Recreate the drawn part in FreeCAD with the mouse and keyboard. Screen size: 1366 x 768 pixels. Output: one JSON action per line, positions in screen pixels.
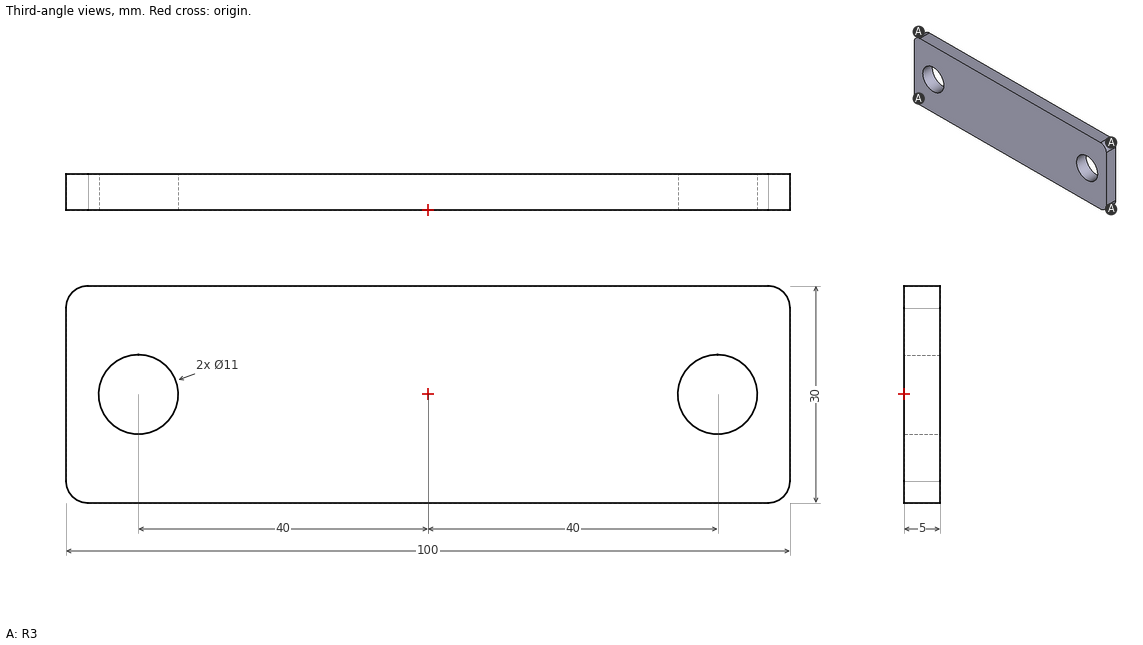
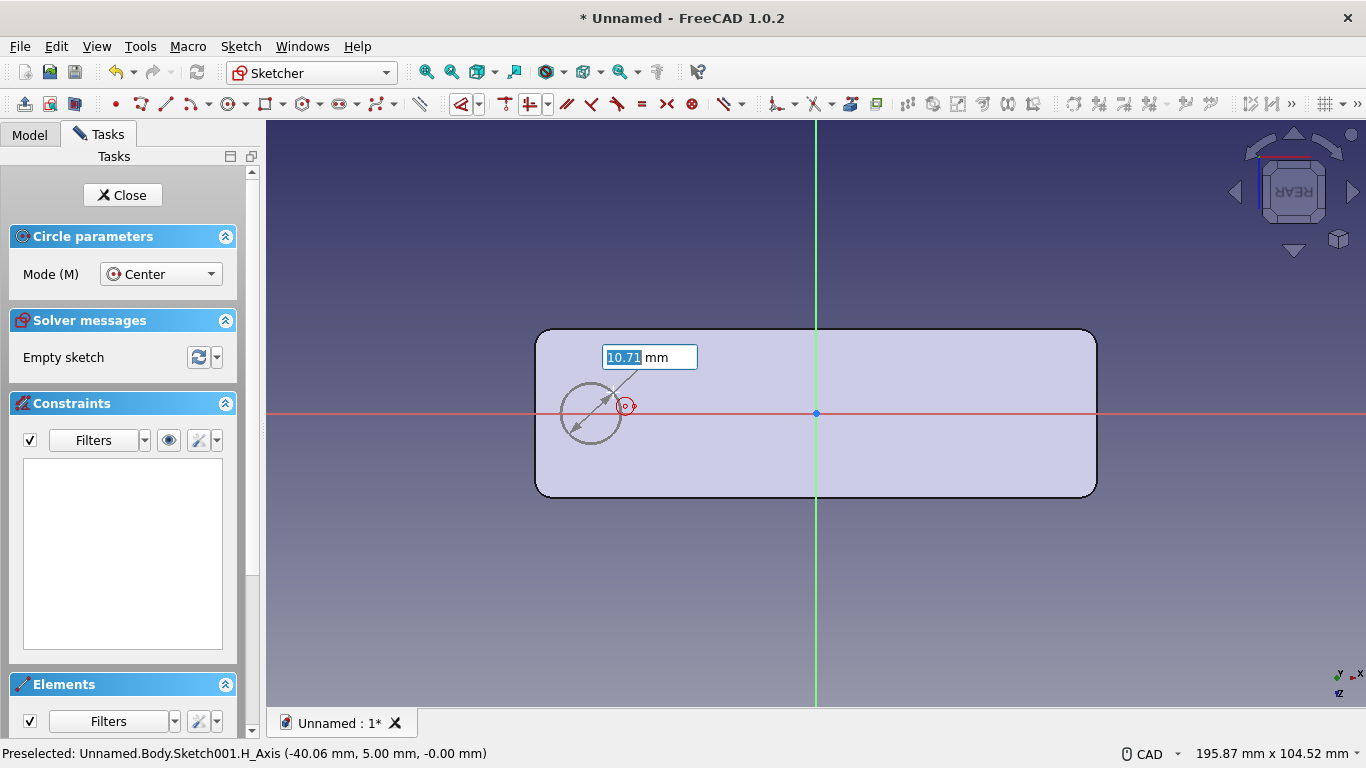
{"action": "type", "text": "11"}
{"action": "key", "text": "Return"}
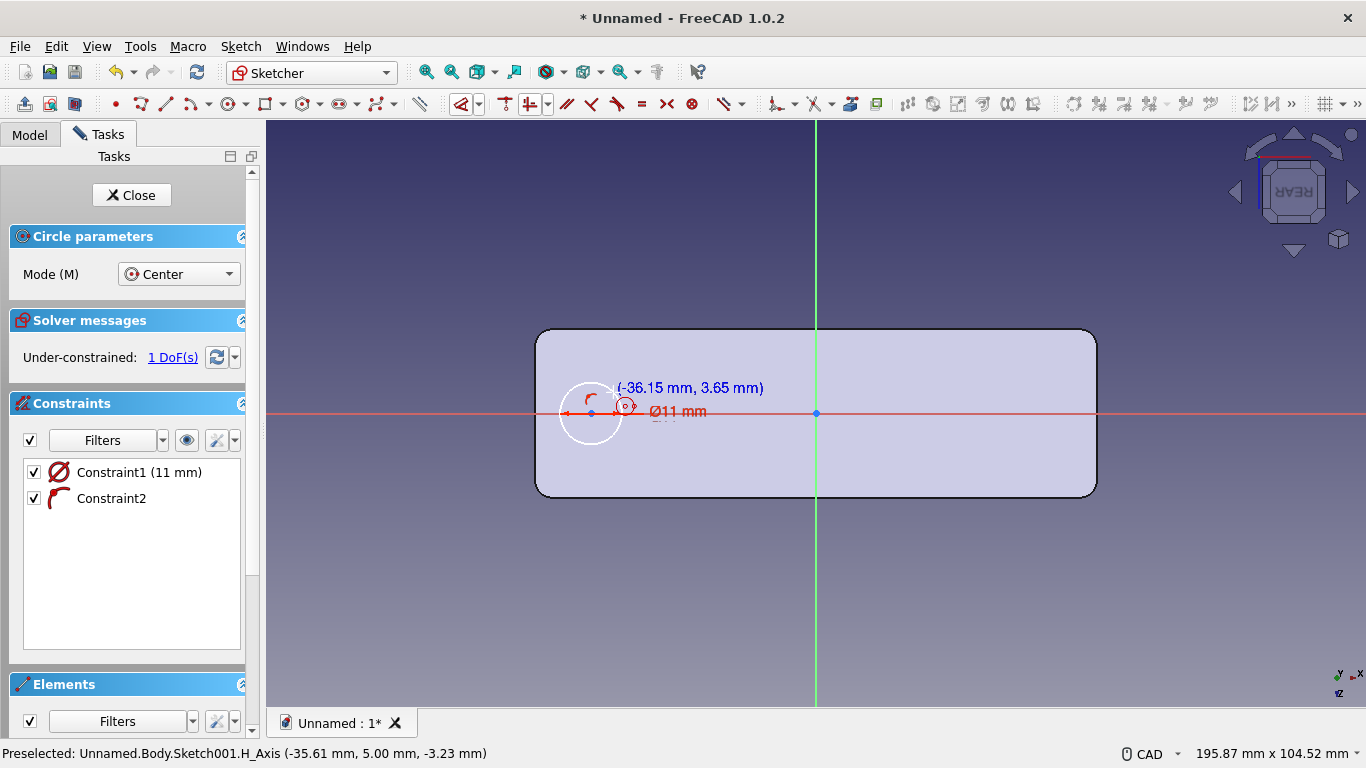
{"action": "left_click", "coordinate": [1041, 414]}
{"action": "mouse_move", "coordinate": [1062, 392]}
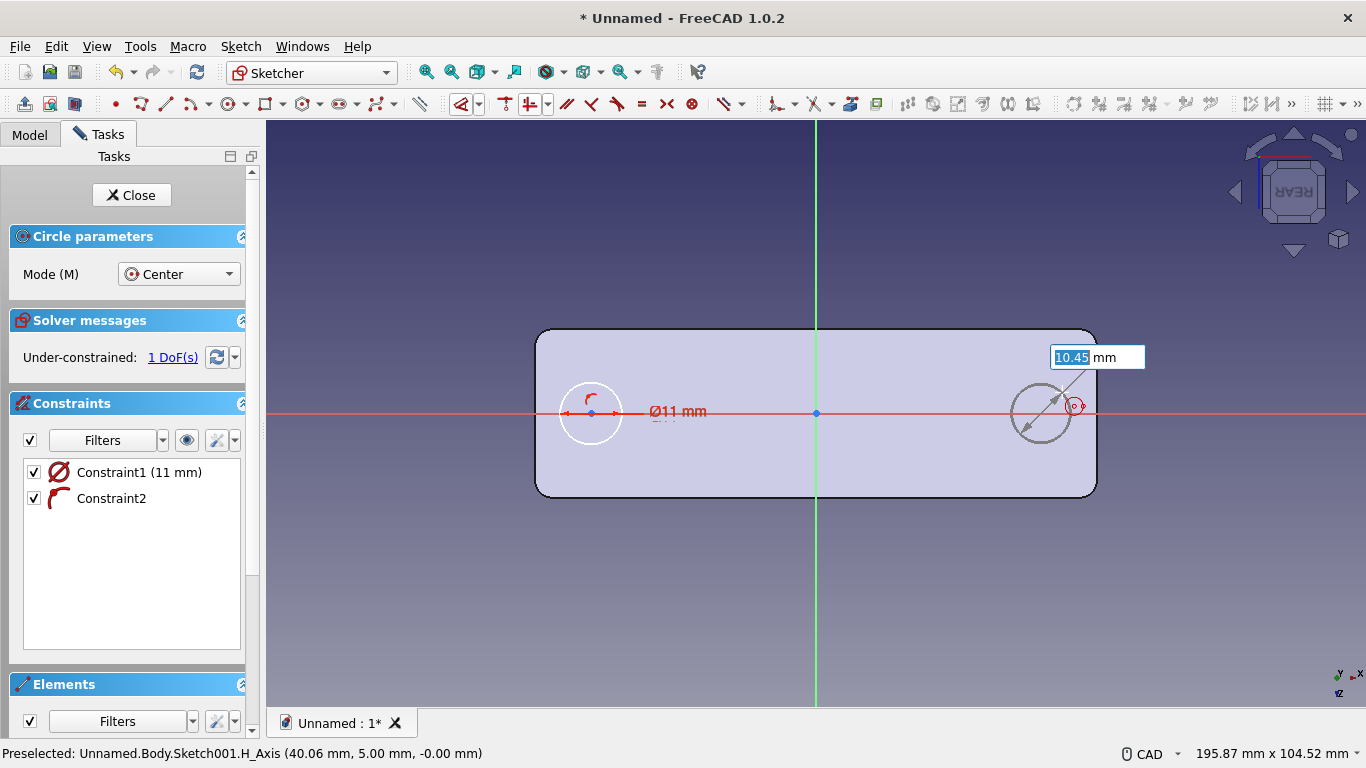
{"action": "type", "text": "11"}
{"action": "key", "text": "Return"}
{"action": "key", "text": "Escape"}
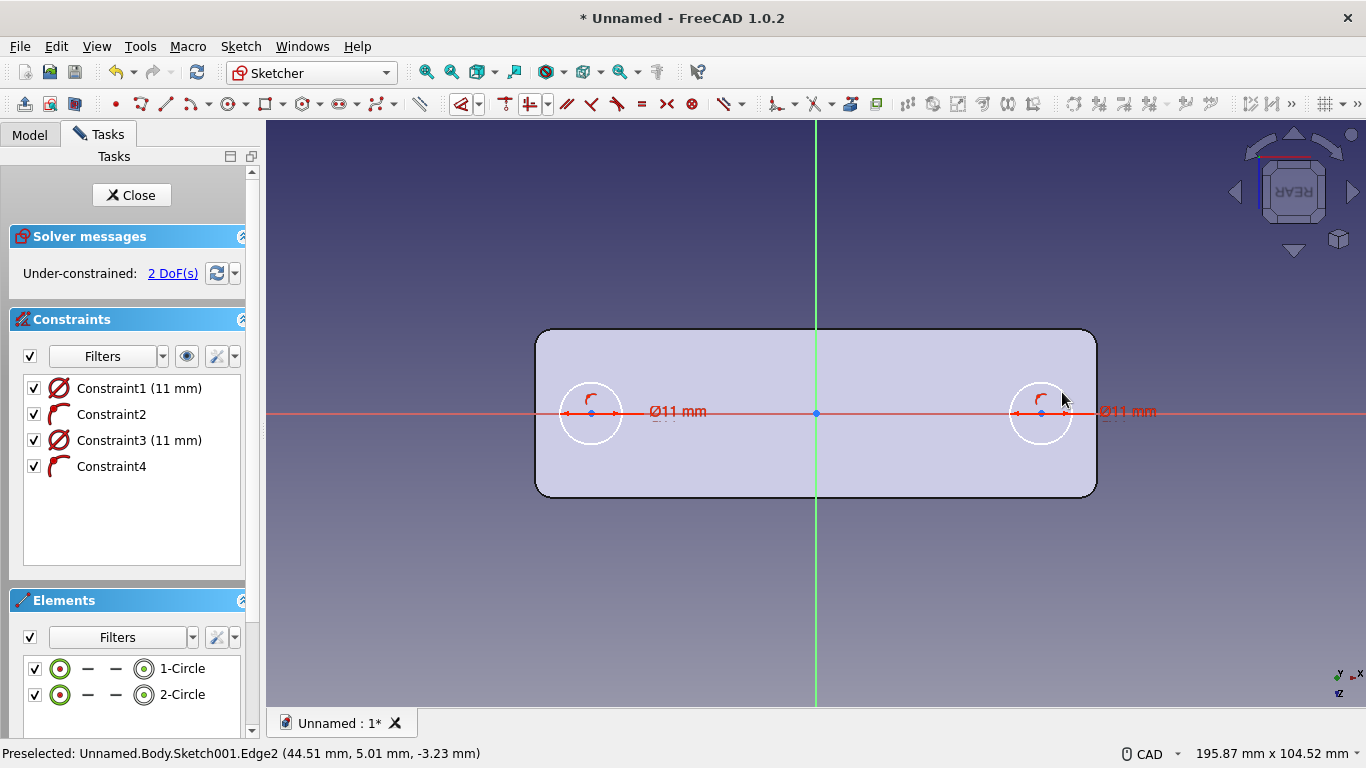
{"action": "key", "text": "d"}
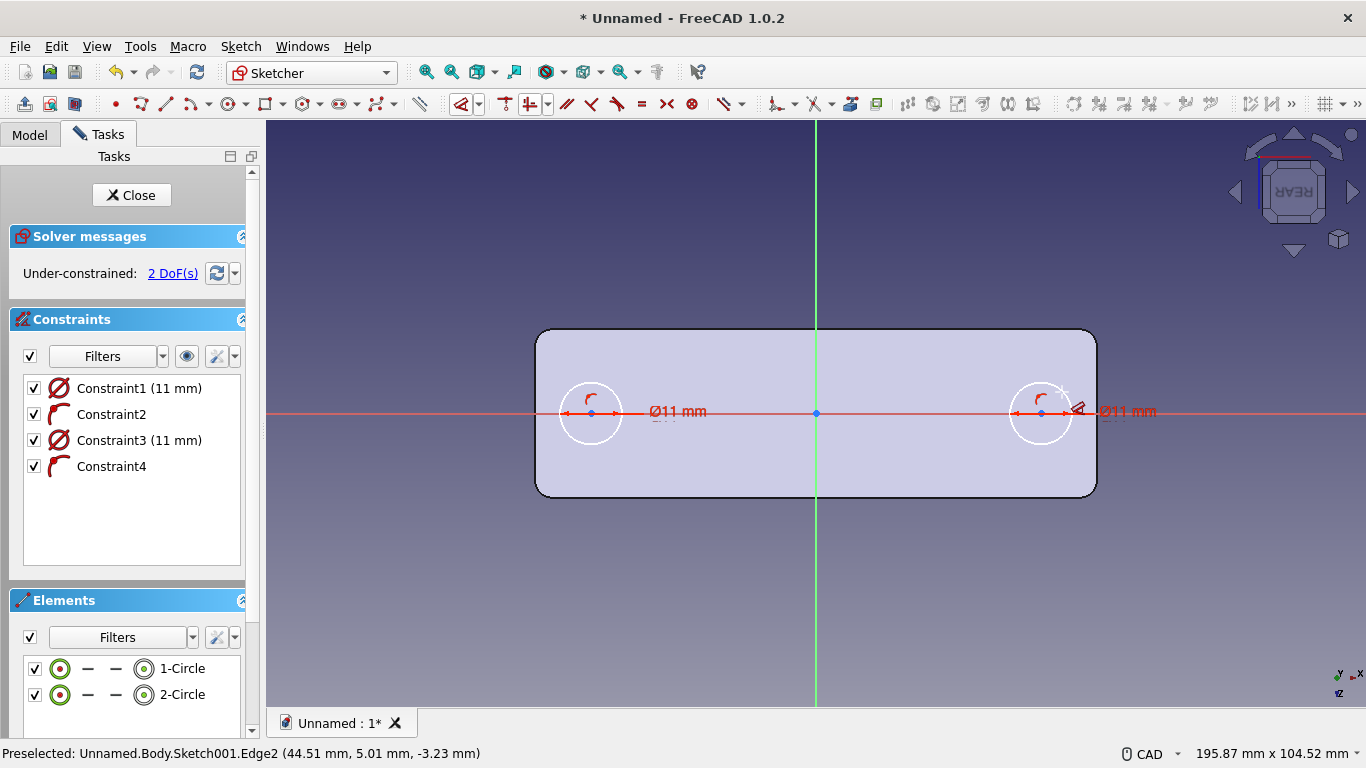
{"action": "left_click", "coordinate": [591, 414]}
{"action": "left_click", "coordinate": [703, 448]}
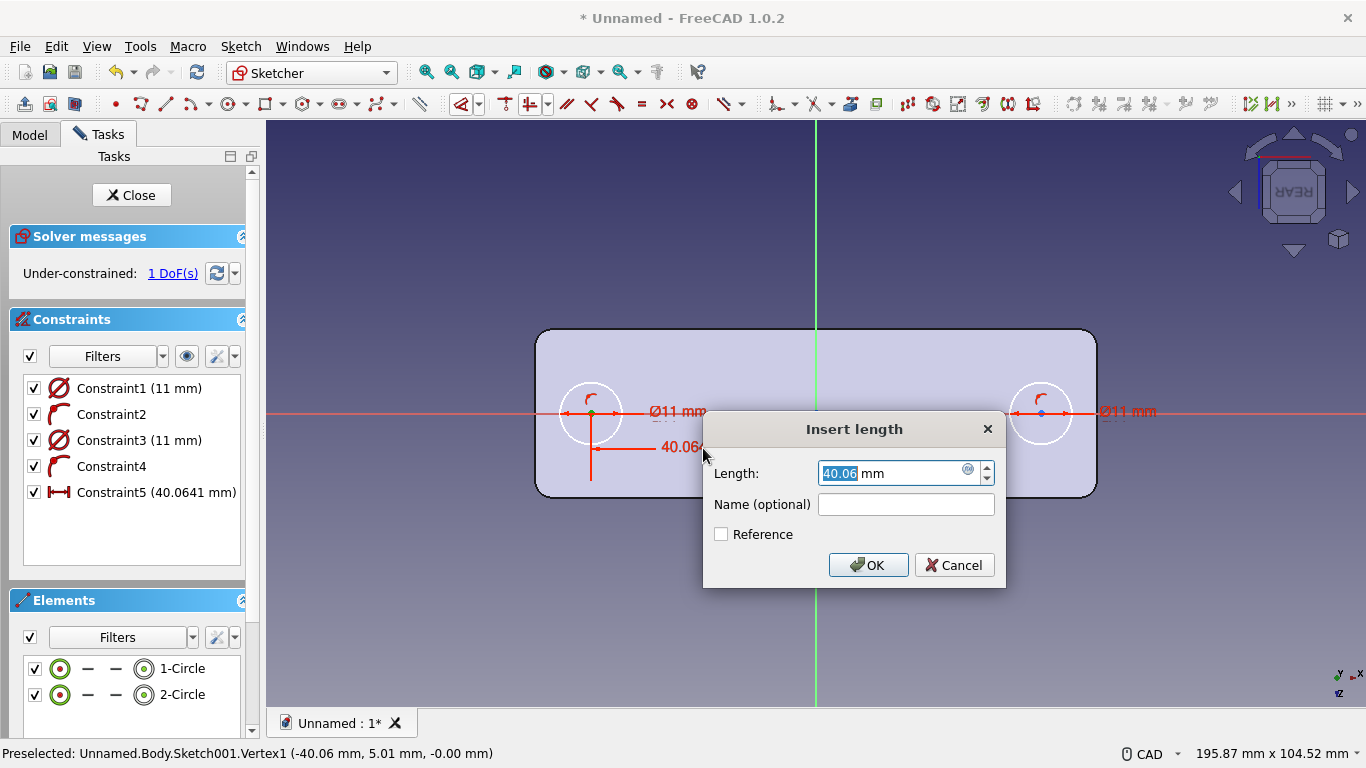
{"action": "type", "text": "40"}
{"action": "key", "text": "Return"}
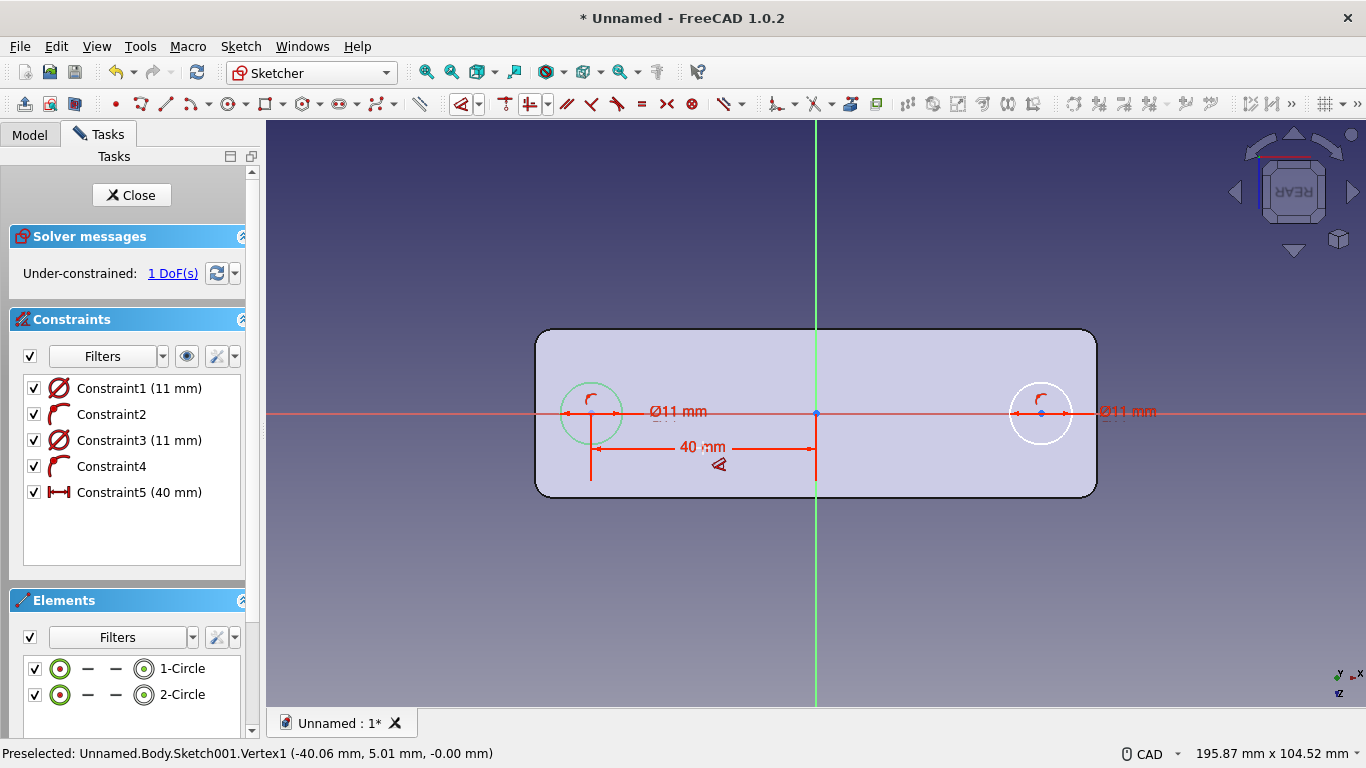
{"action": "left_click", "coordinate": [1041, 414]}
{"action": "left_click", "coordinate": [928, 448]}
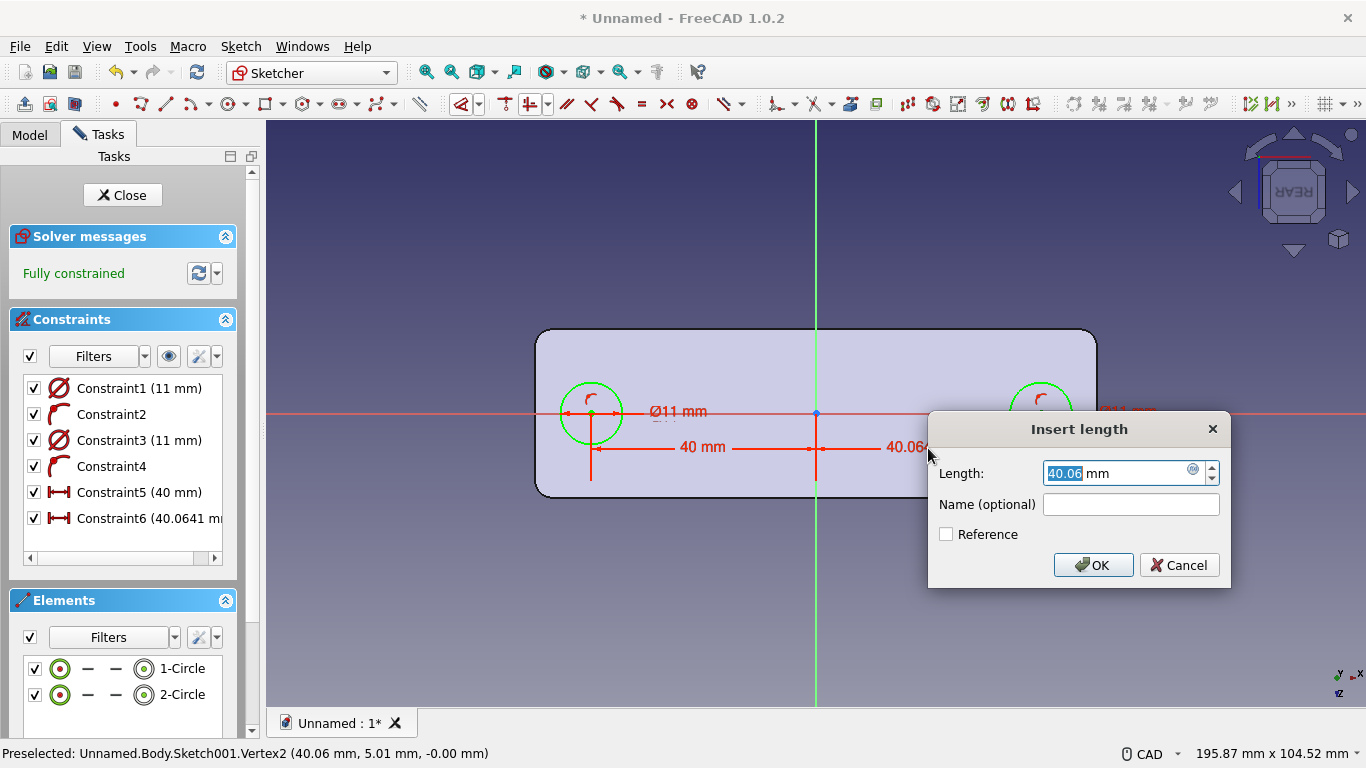
{"action": "type", "text": "40"}
{"action": "key", "text": "Return"}
{"action": "key", "text": "Escape"}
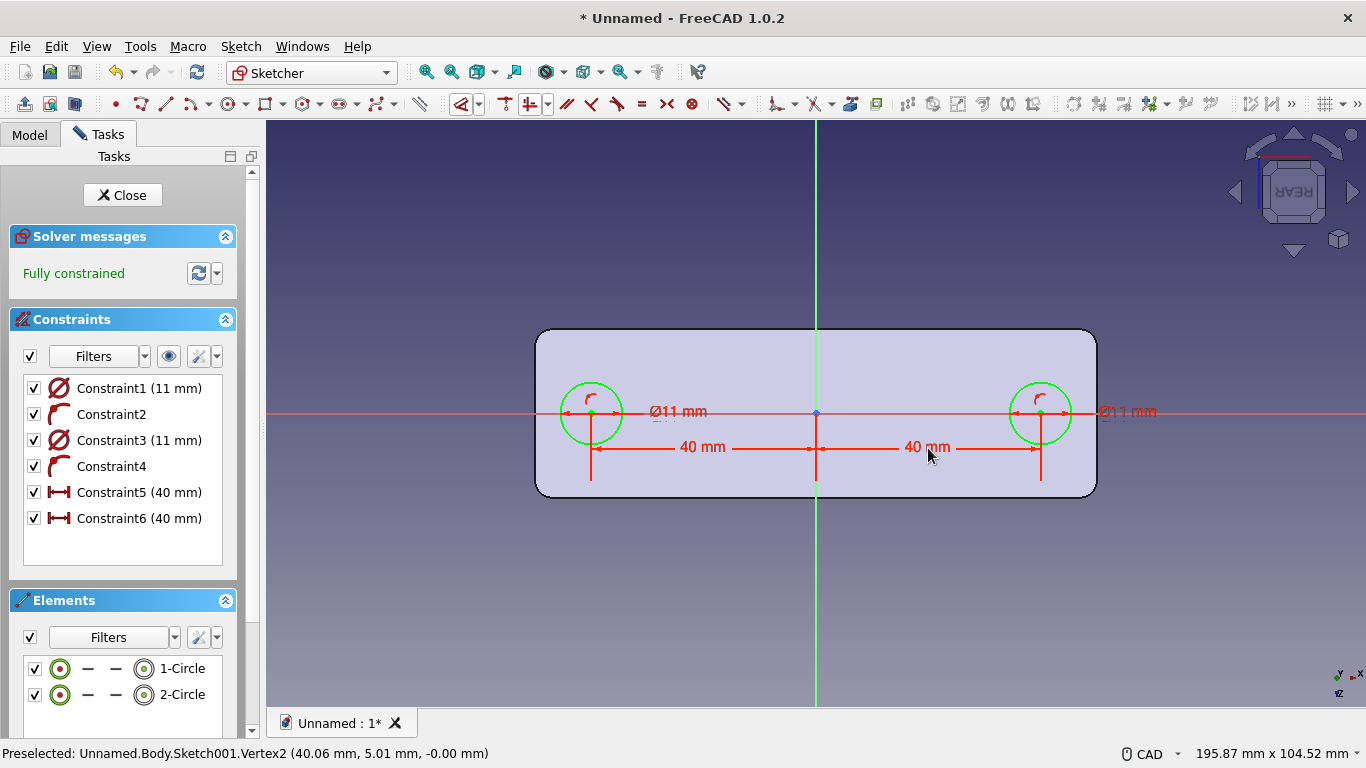
{"action": "left_click", "coordinate": [123, 195]}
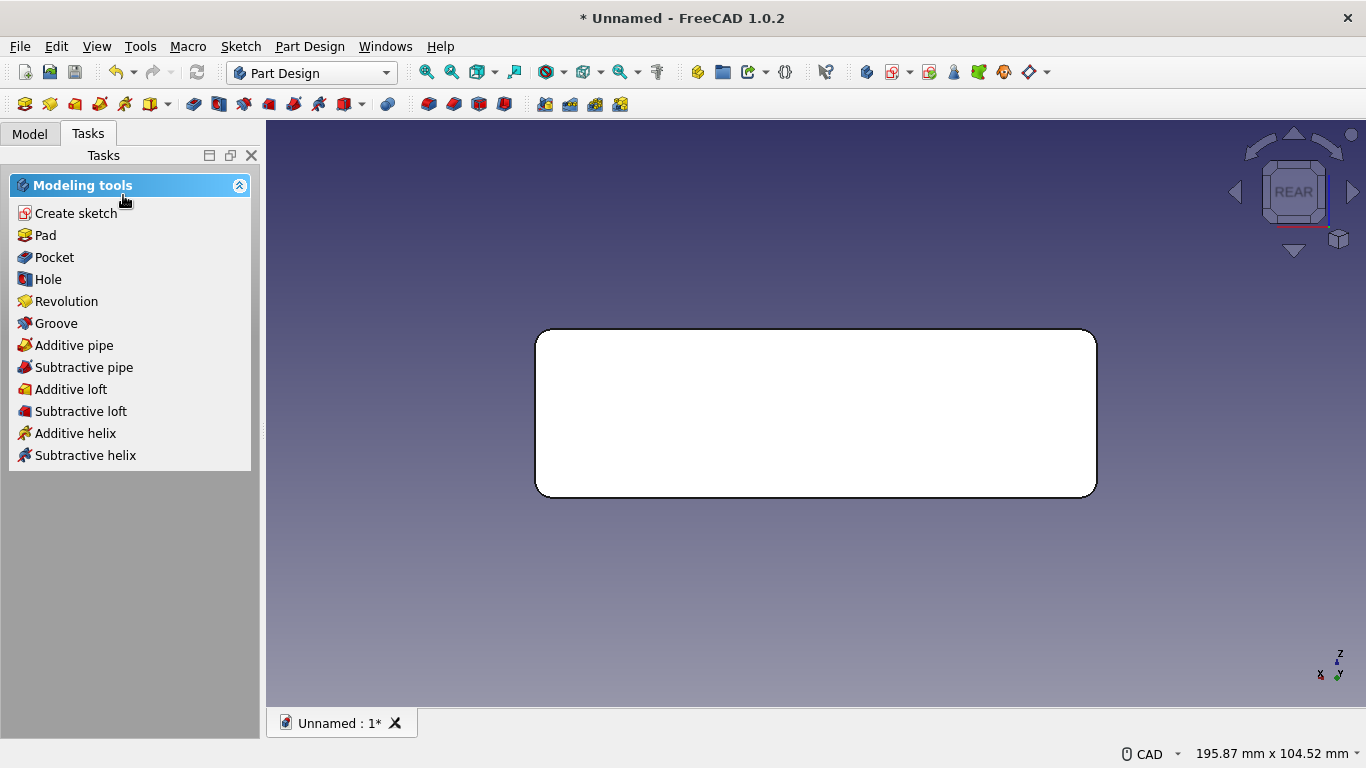
{"action": "left_click", "coordinate": [194, 104]}